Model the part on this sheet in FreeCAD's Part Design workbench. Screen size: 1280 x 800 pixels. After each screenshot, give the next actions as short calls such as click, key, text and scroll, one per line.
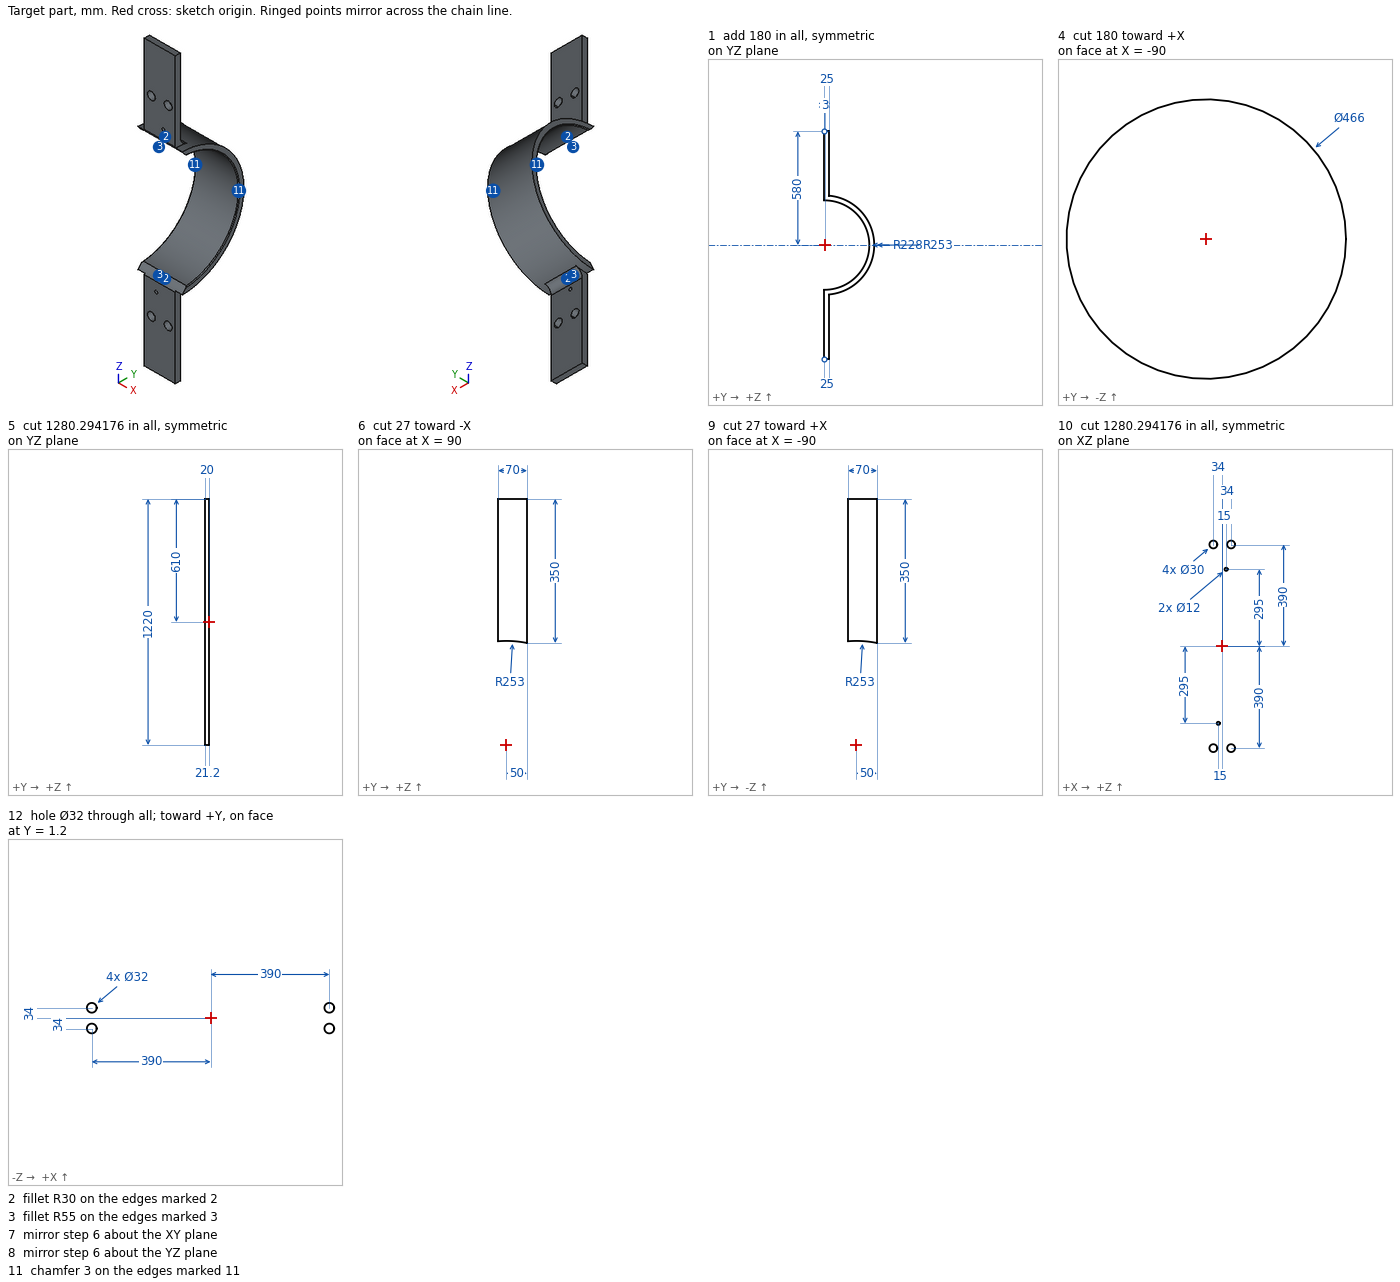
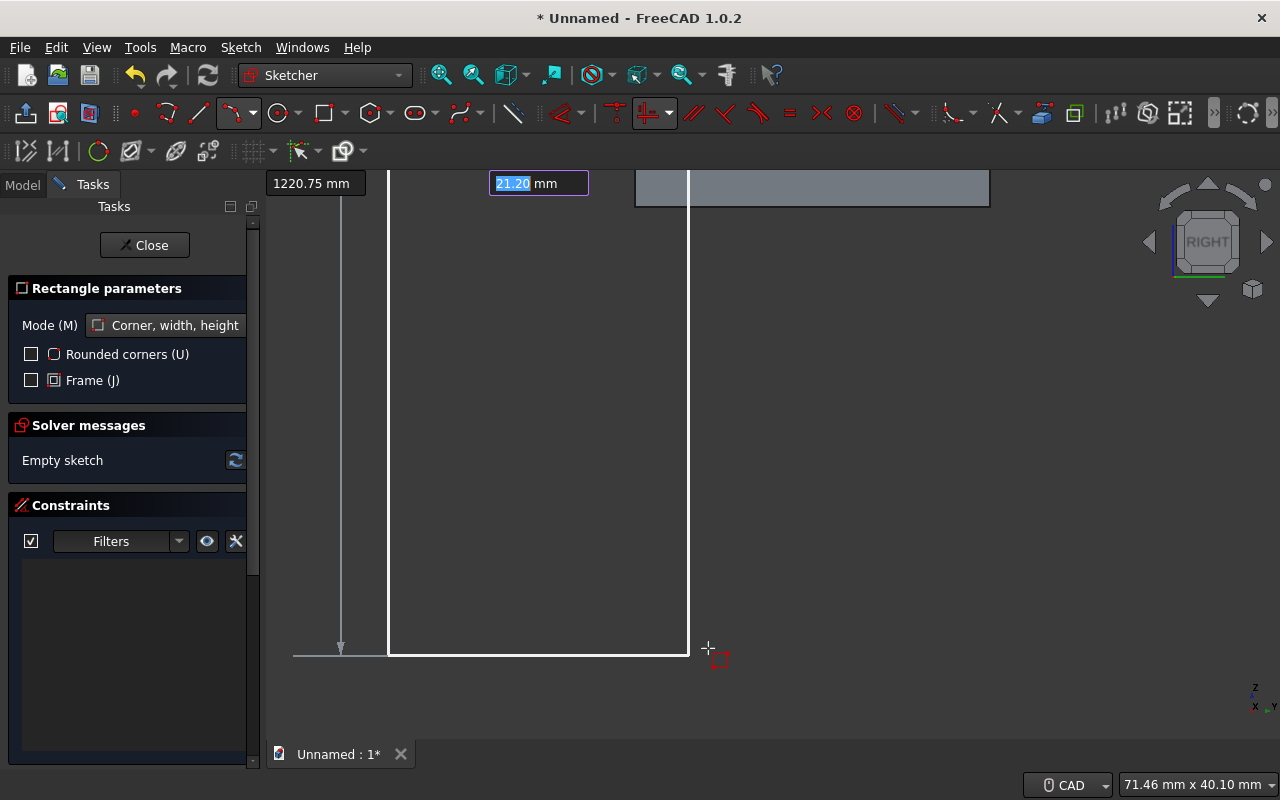
click(694, 633)
key(Escape)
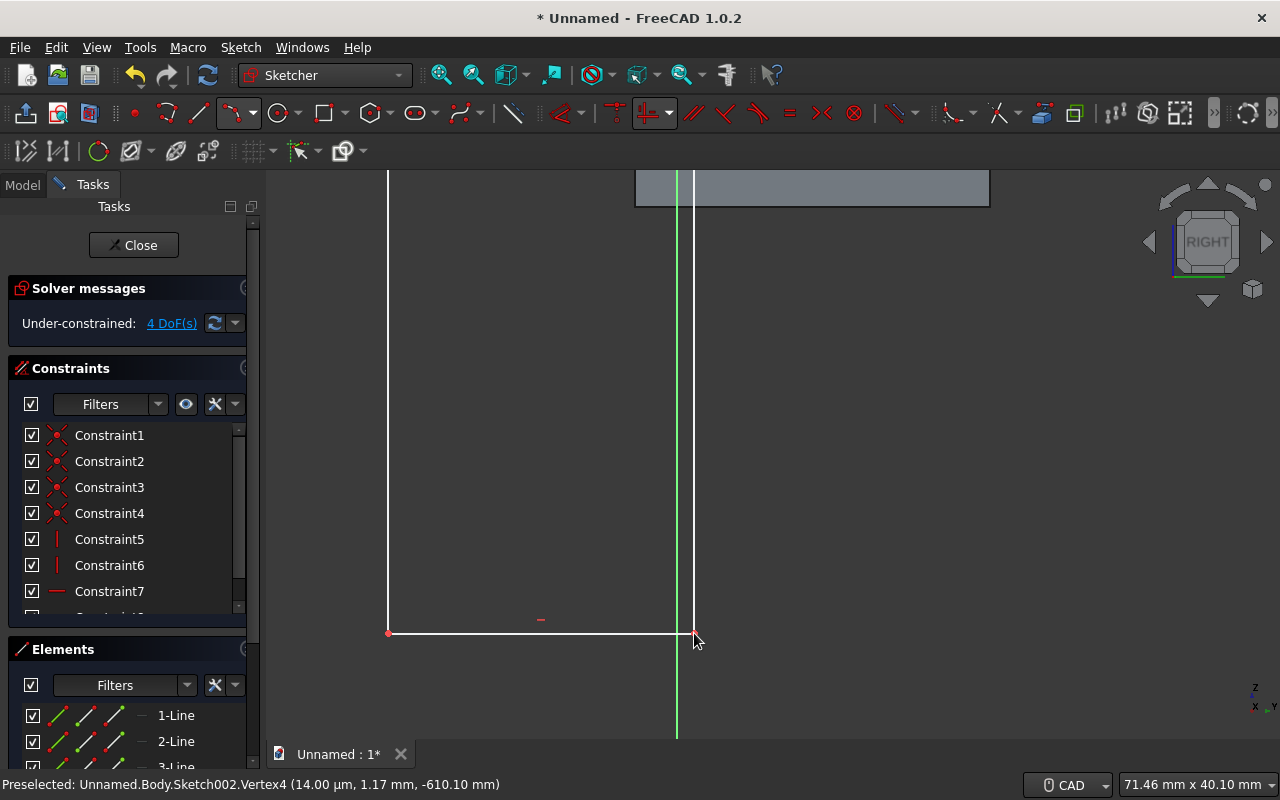
click(560, 114)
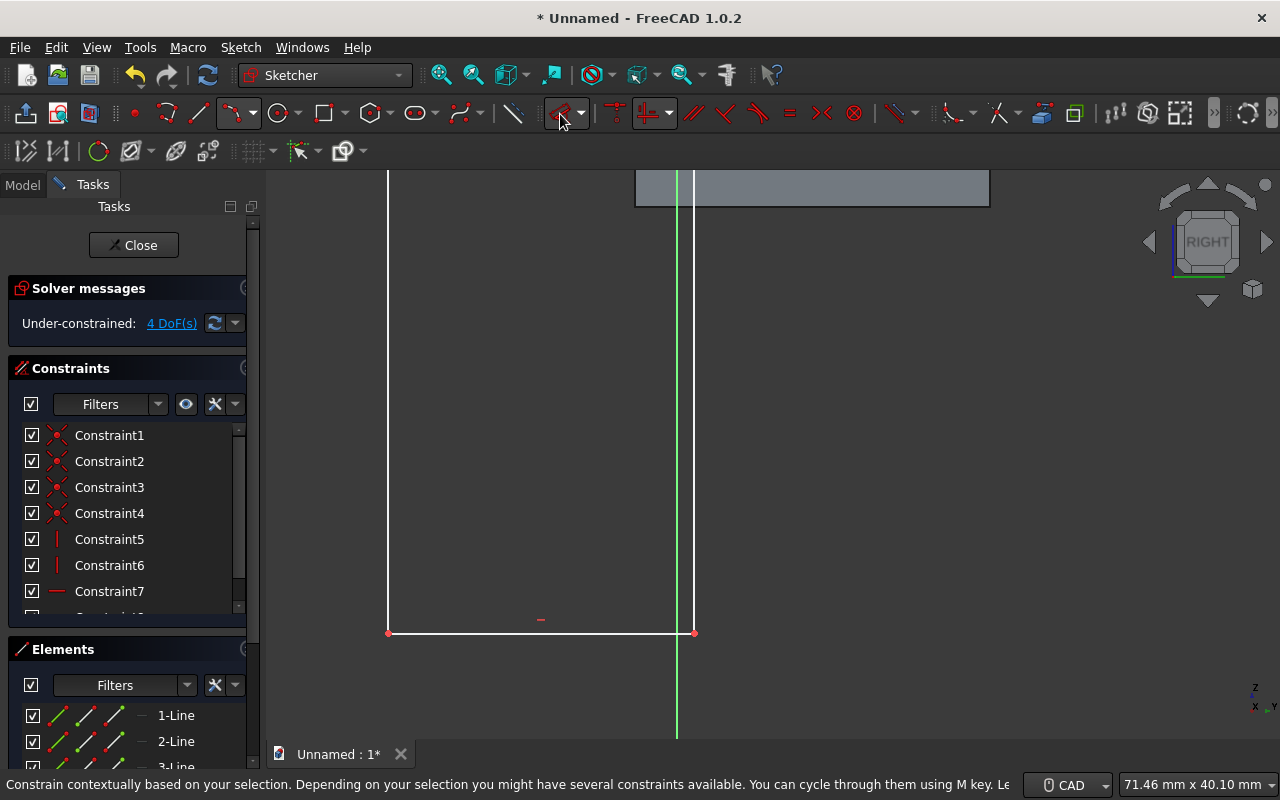
scroll(704, 454, down, 15)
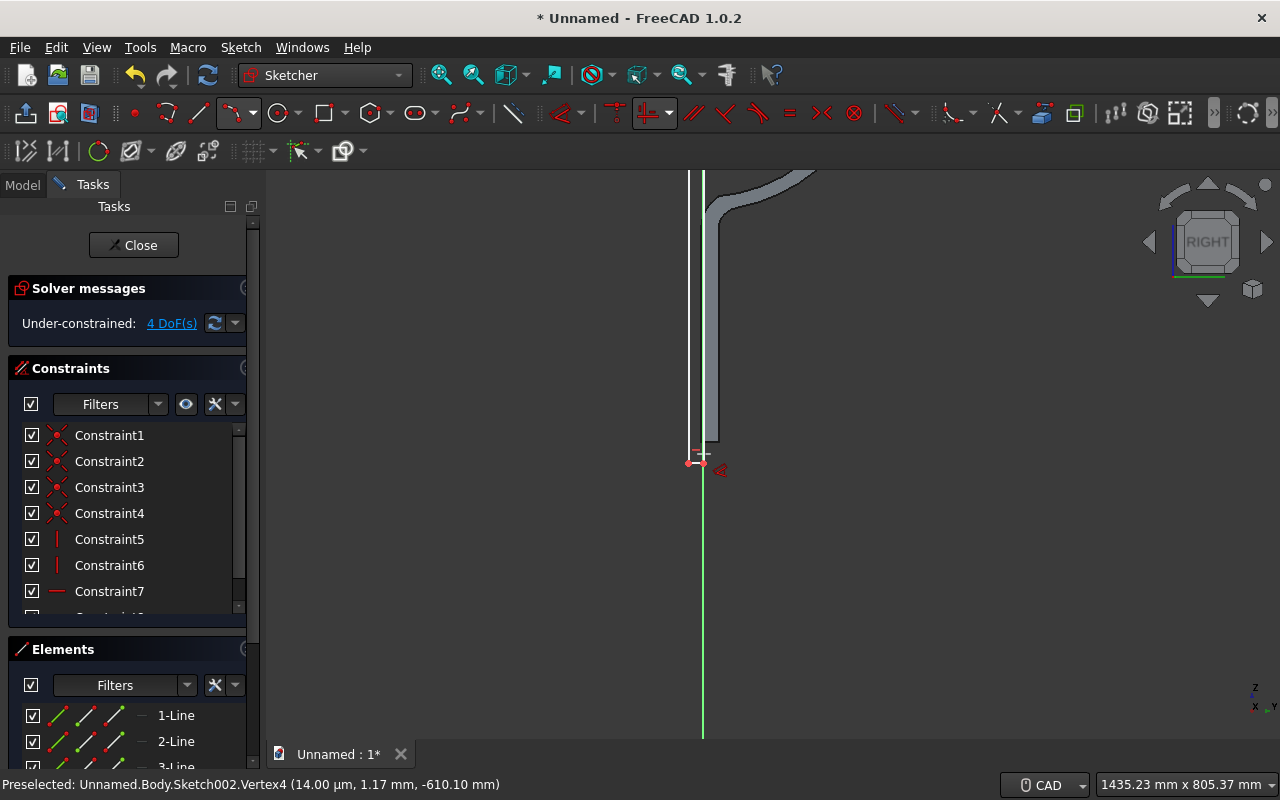
scroll(709, 700, down, 5)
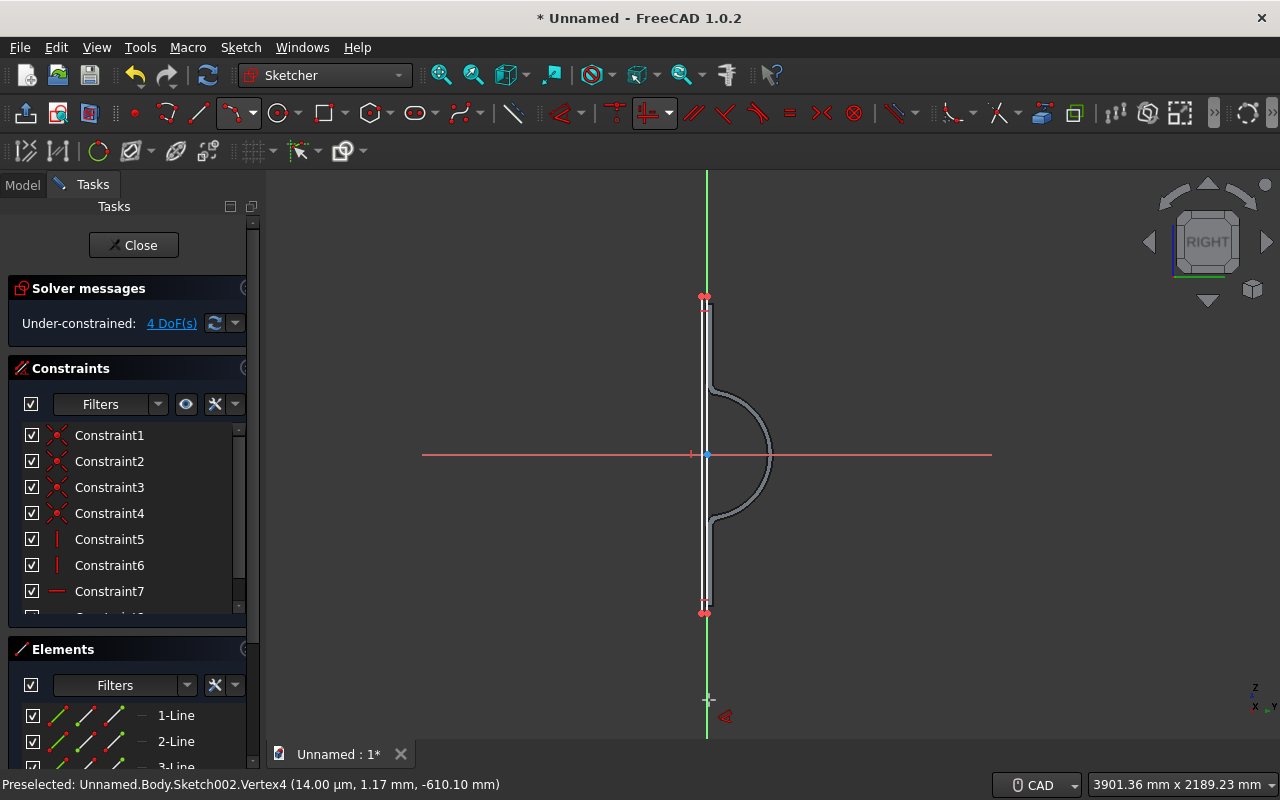
scroll(702, 297, up, 11)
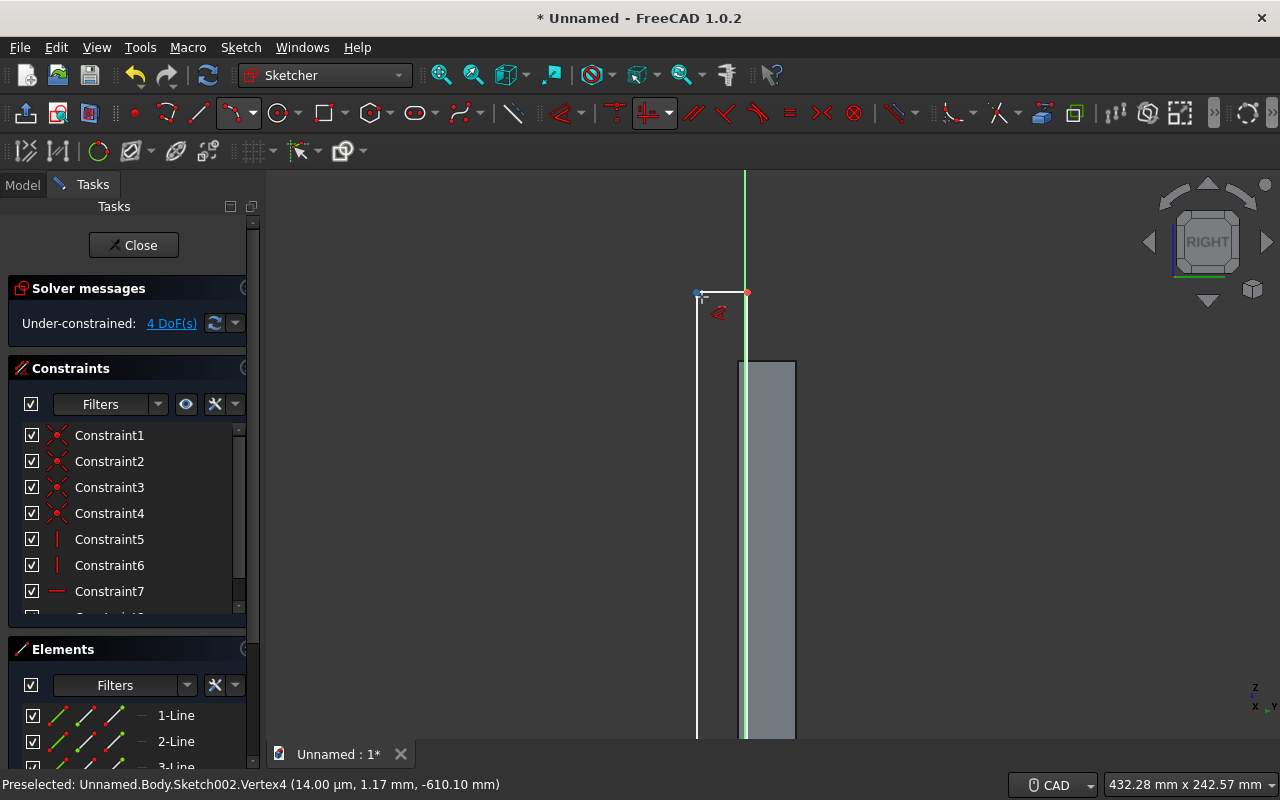
click(697, 292)
click(721, 258)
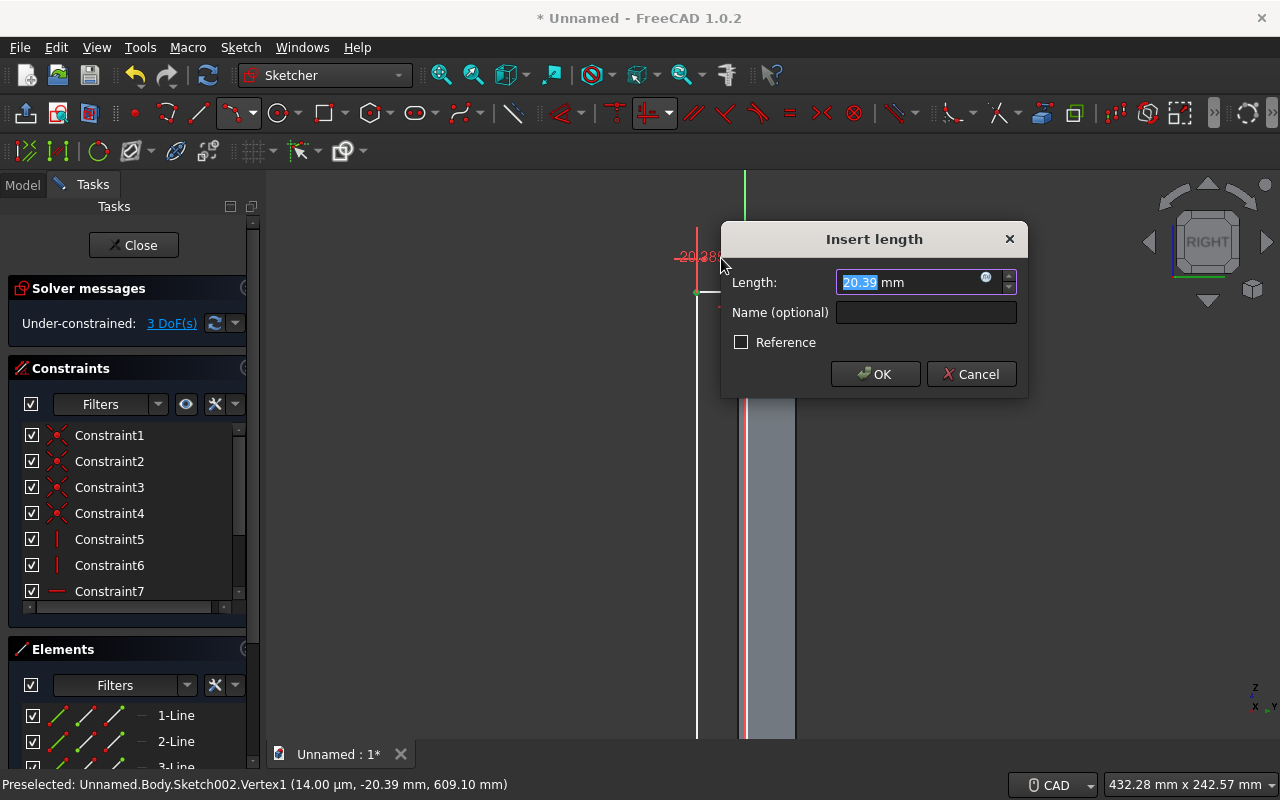
text(20)
key(Return)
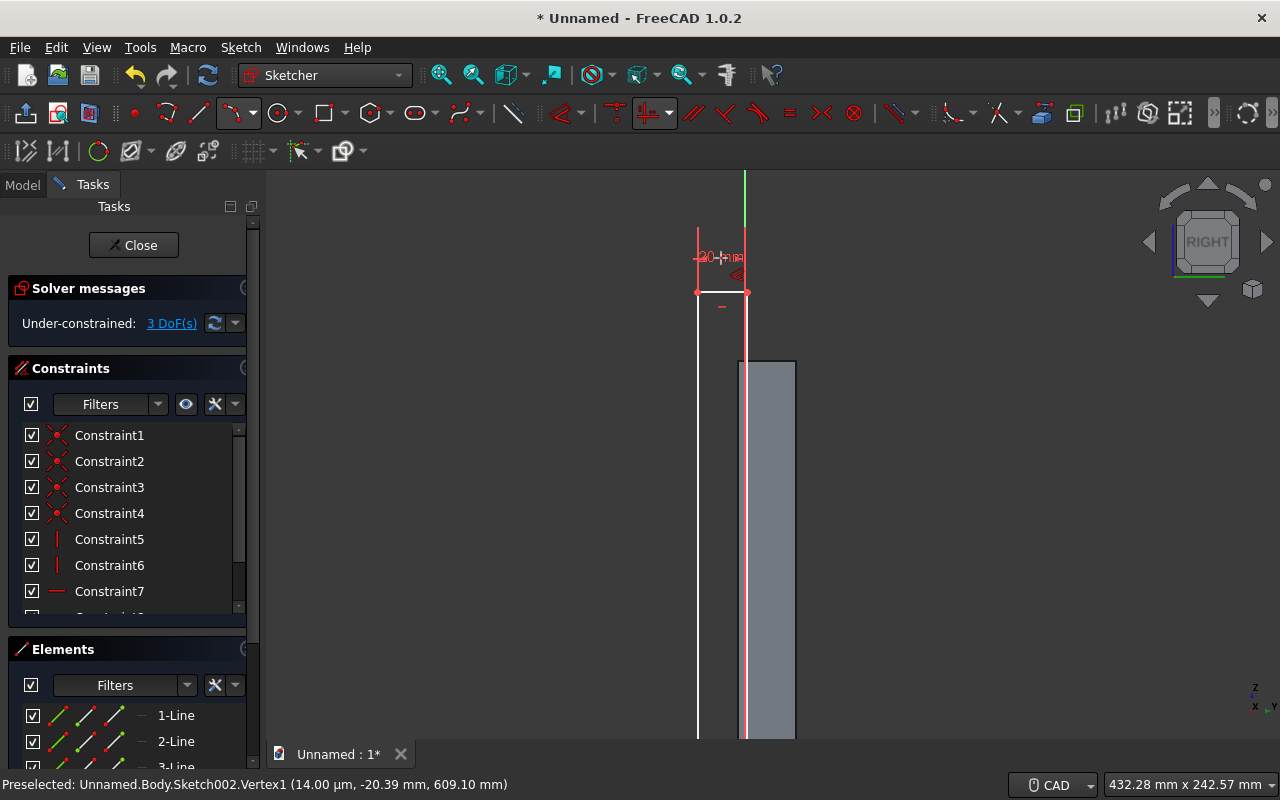
scroll(702, 256, down, 10)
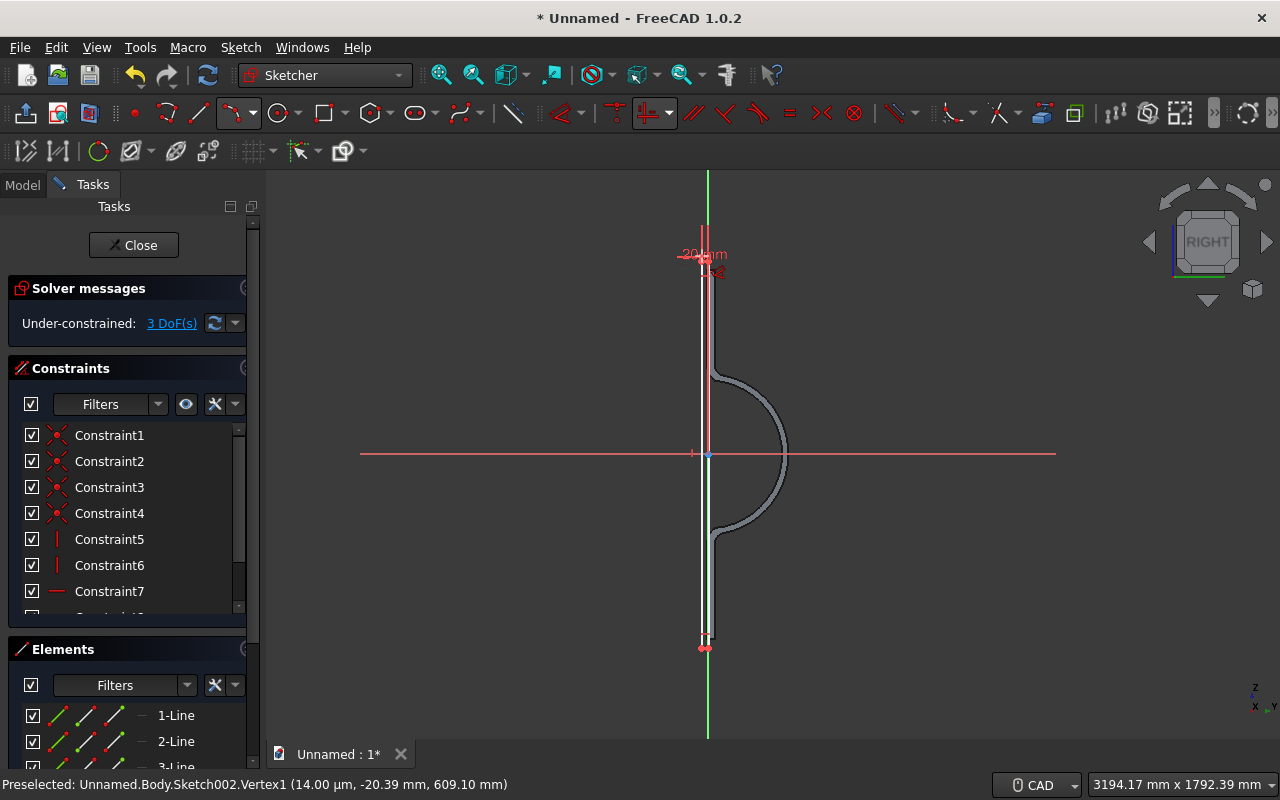
scroll(702, 377, up, 4)